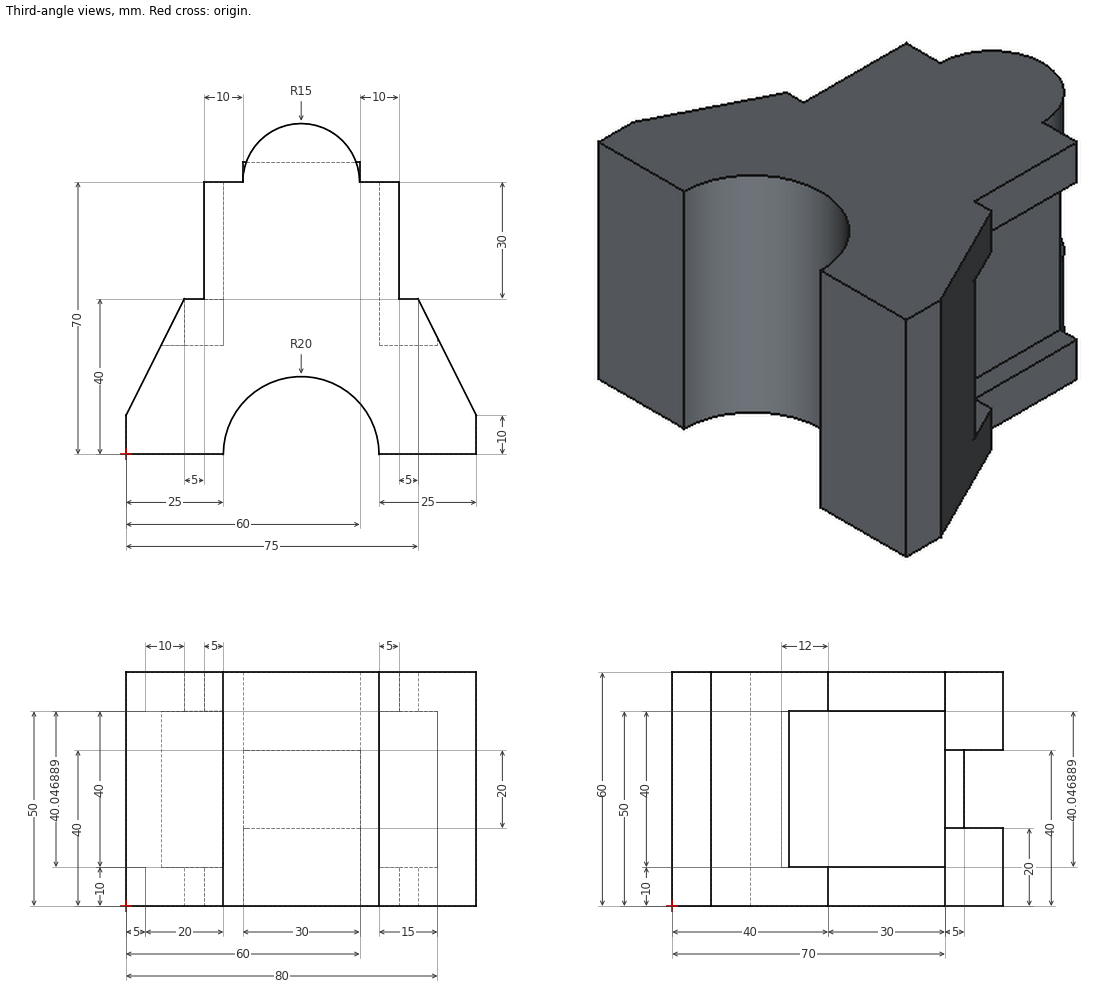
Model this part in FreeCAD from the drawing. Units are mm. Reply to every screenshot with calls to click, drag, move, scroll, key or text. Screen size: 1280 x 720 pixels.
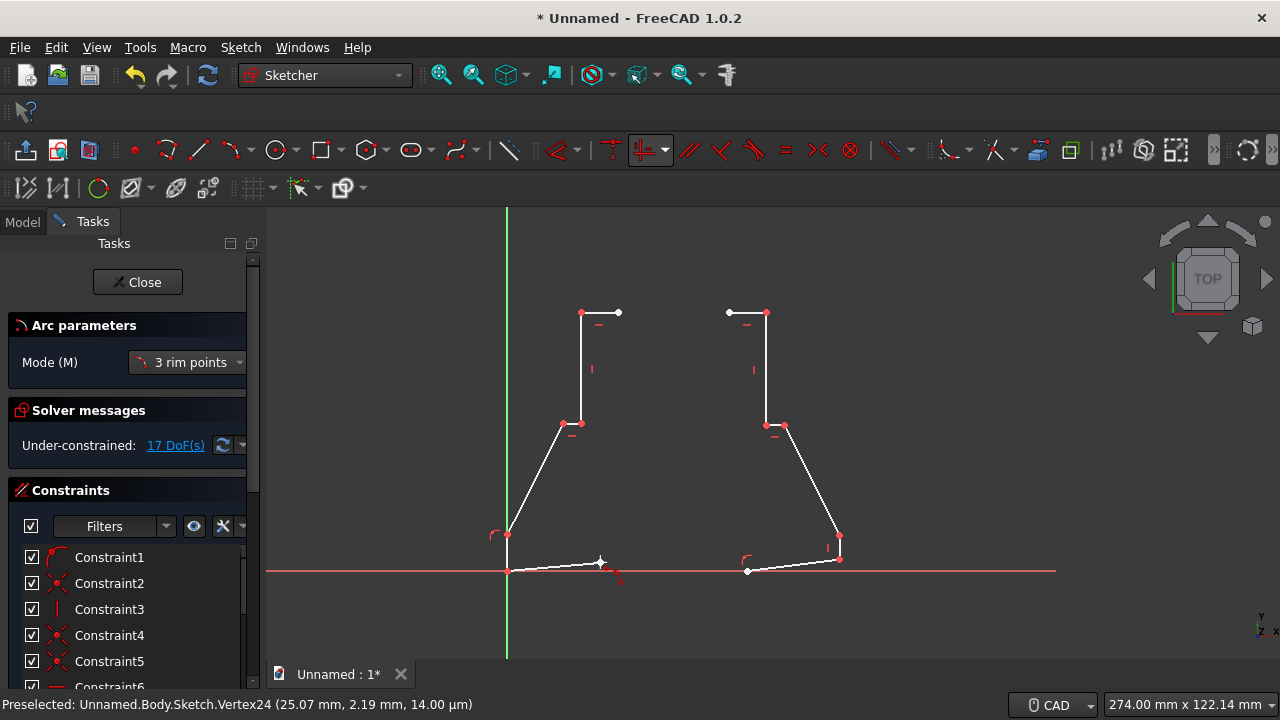
click(729, 313)
click(618, 313)
click(674, 257)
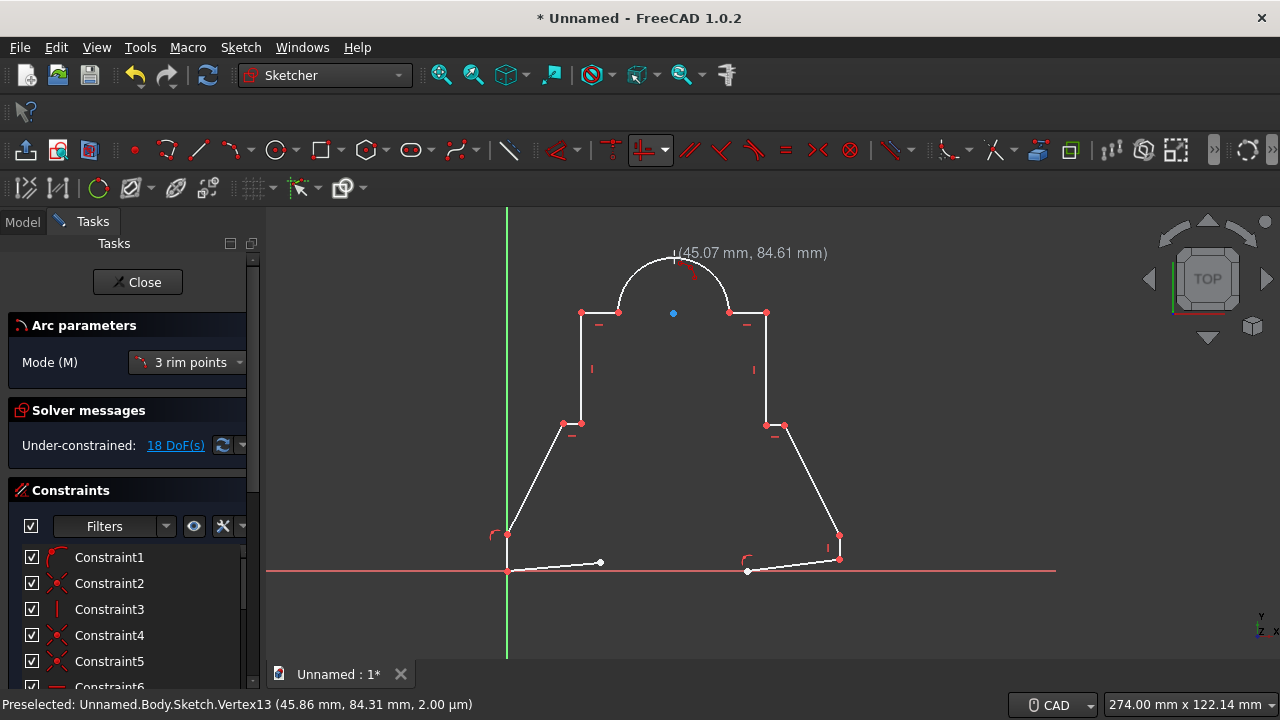
click(600, 563)
click(747, 571)
click(674, 497)
key(Escape)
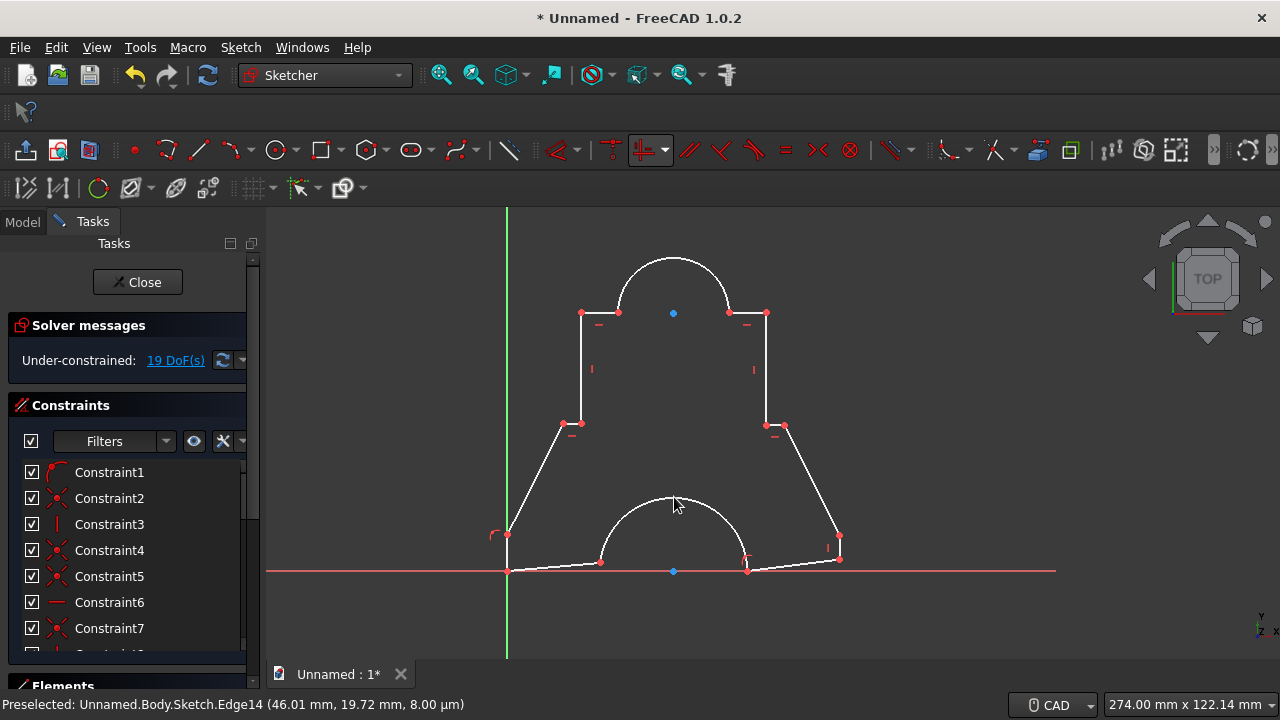
click(775, 568)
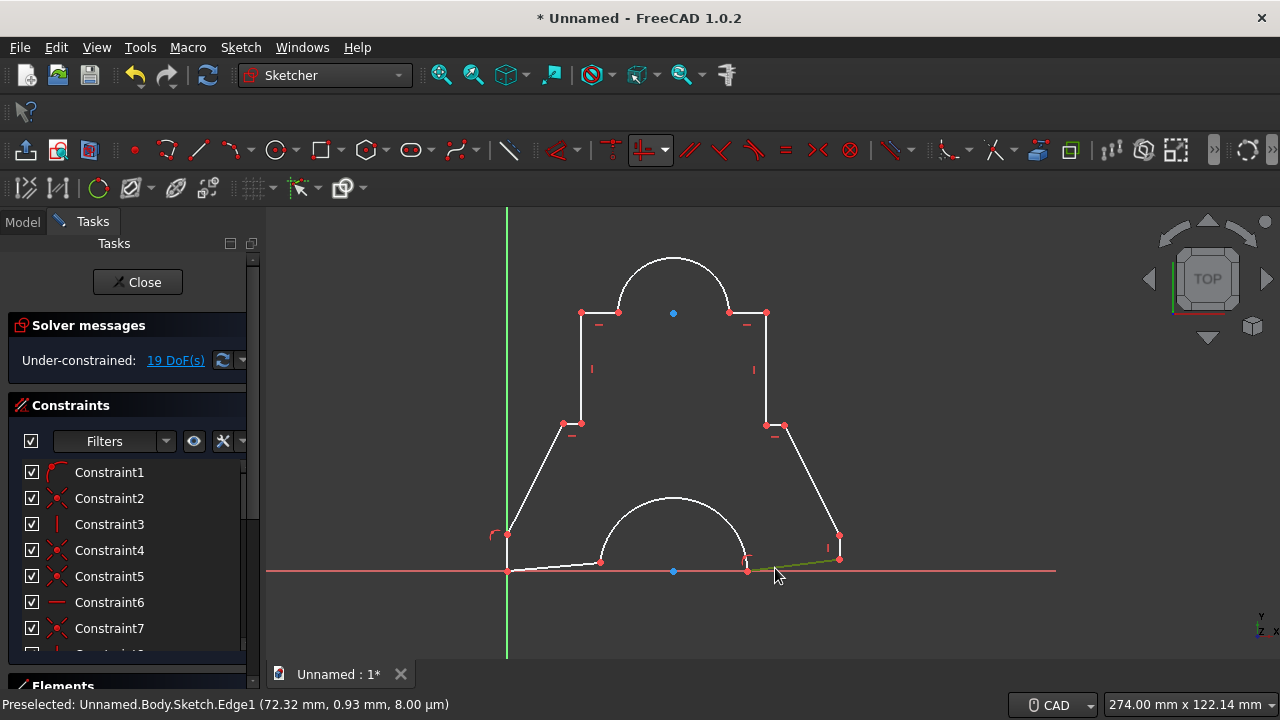
key(h)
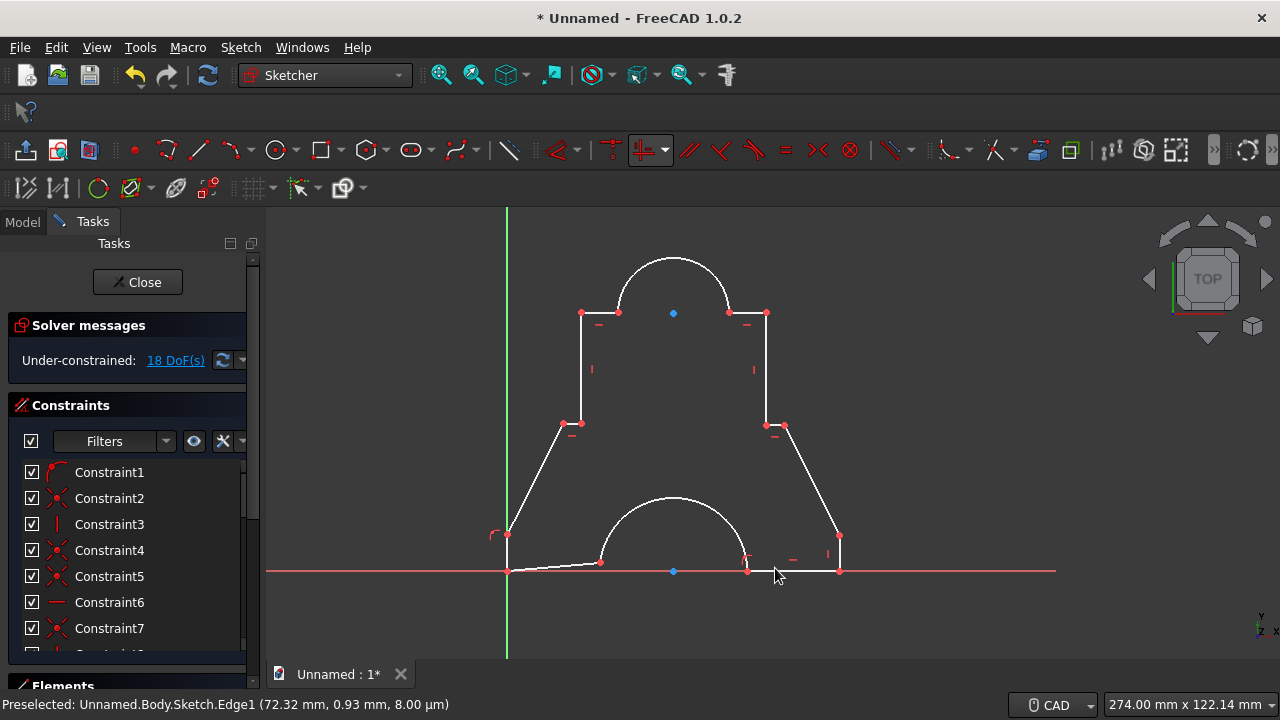
click(535, 569)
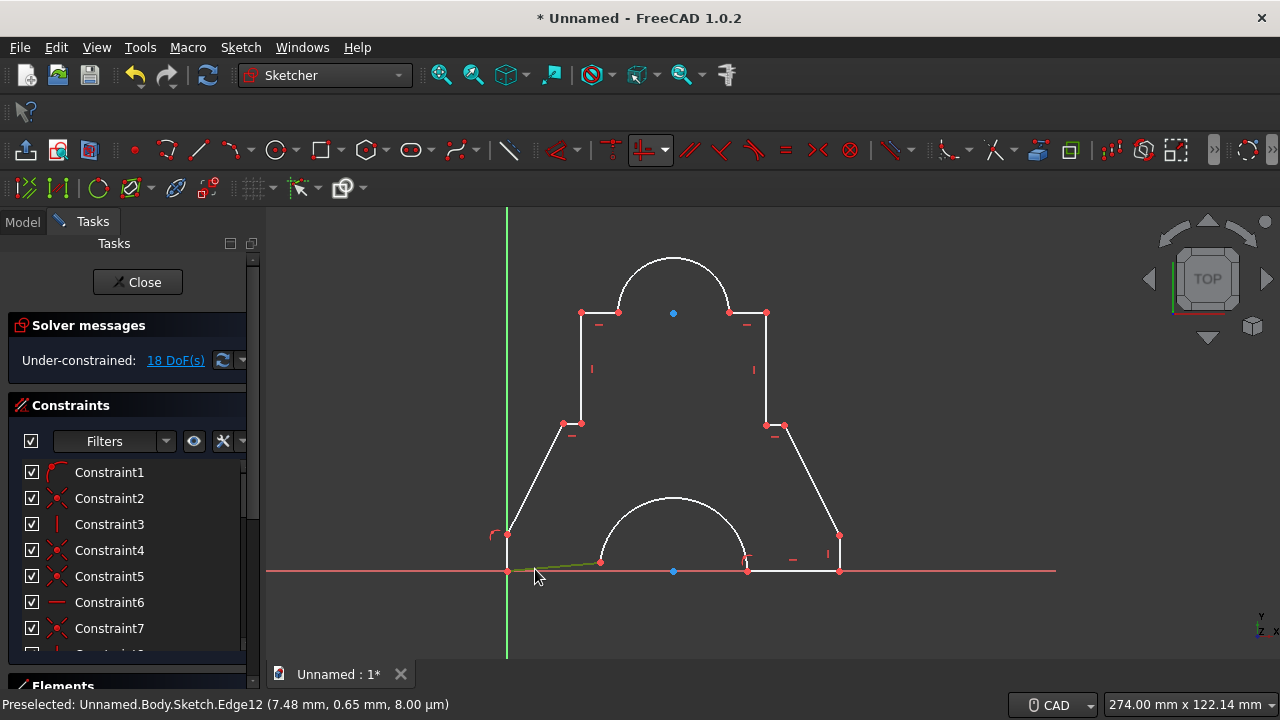
key(h)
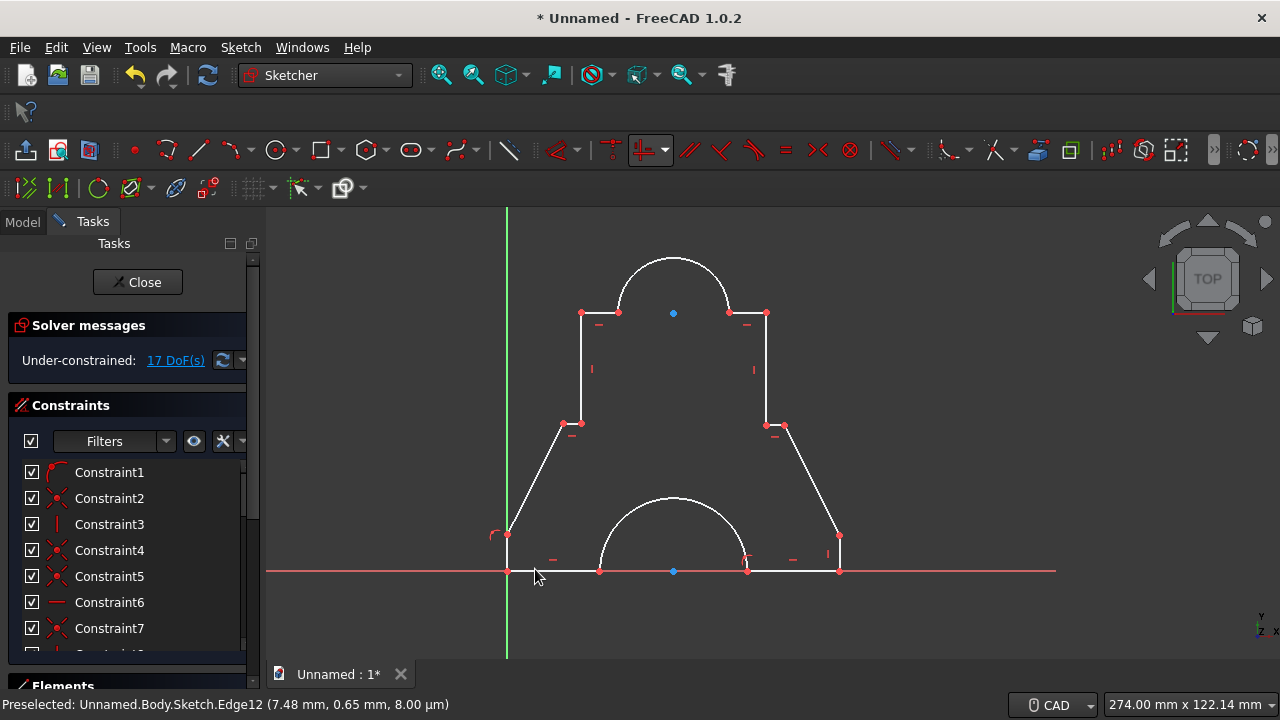
click(674, 572)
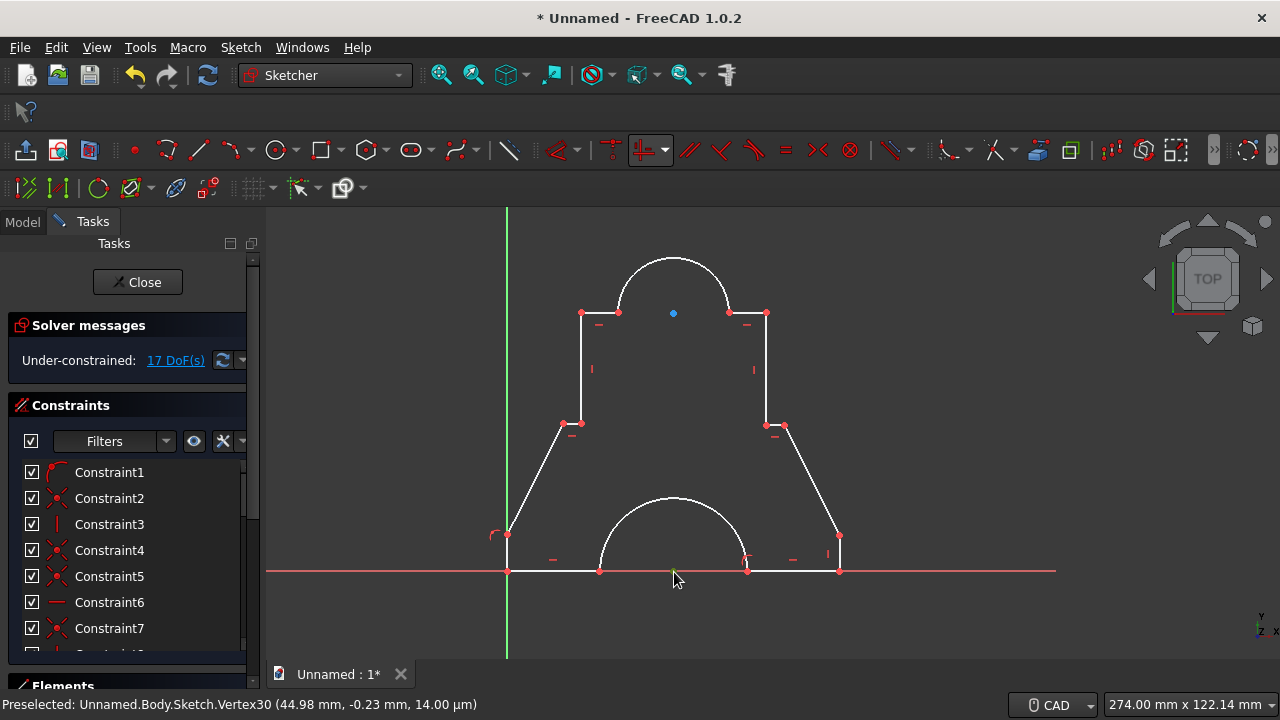
click(353, 571)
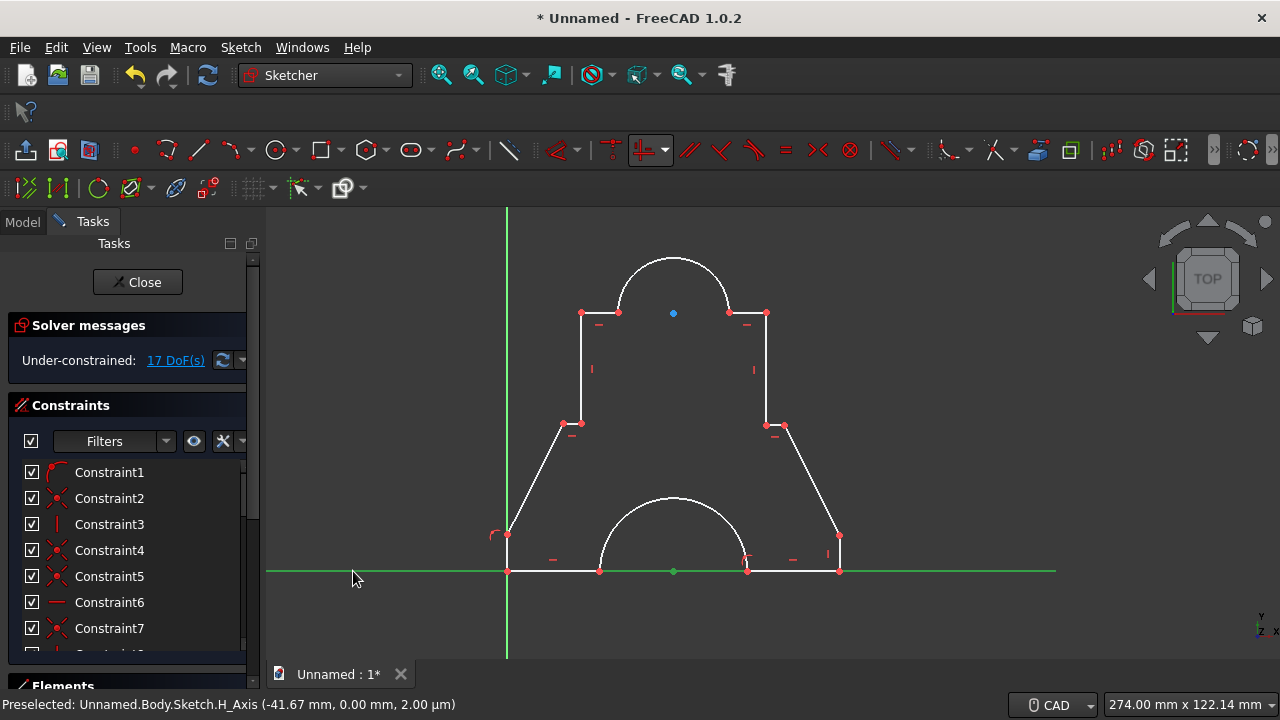
key(c)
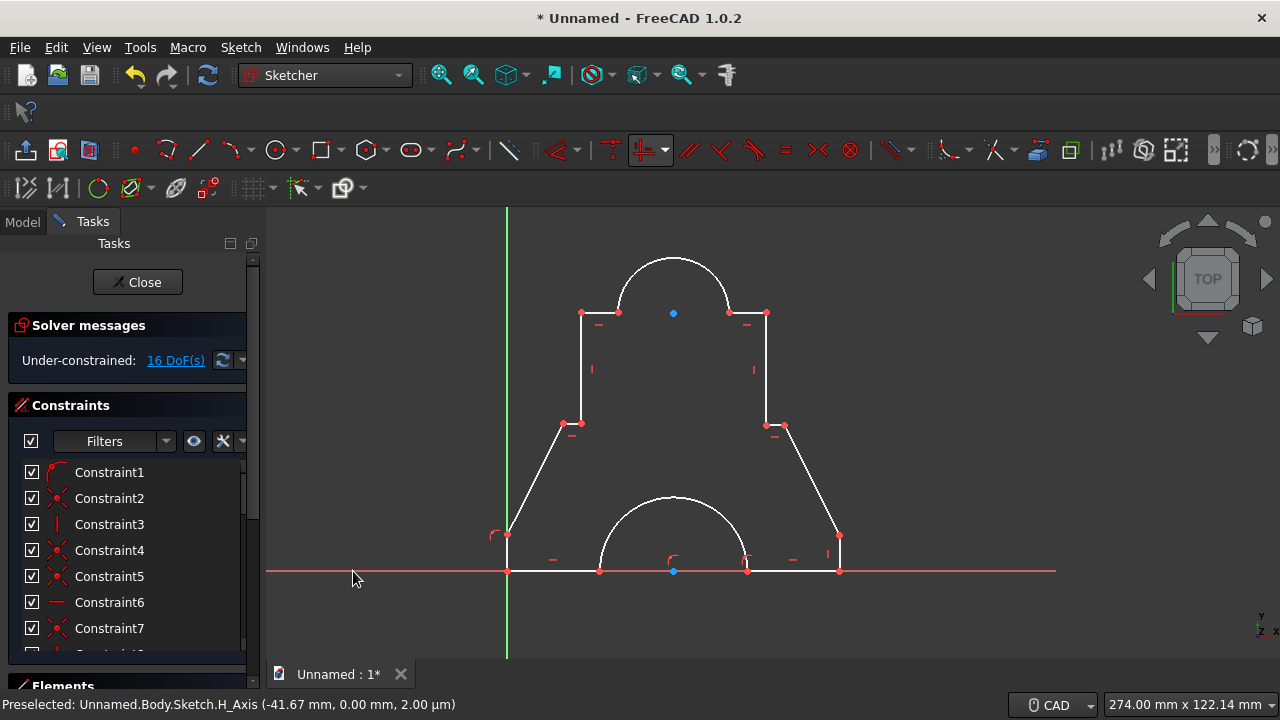
click(556, 150)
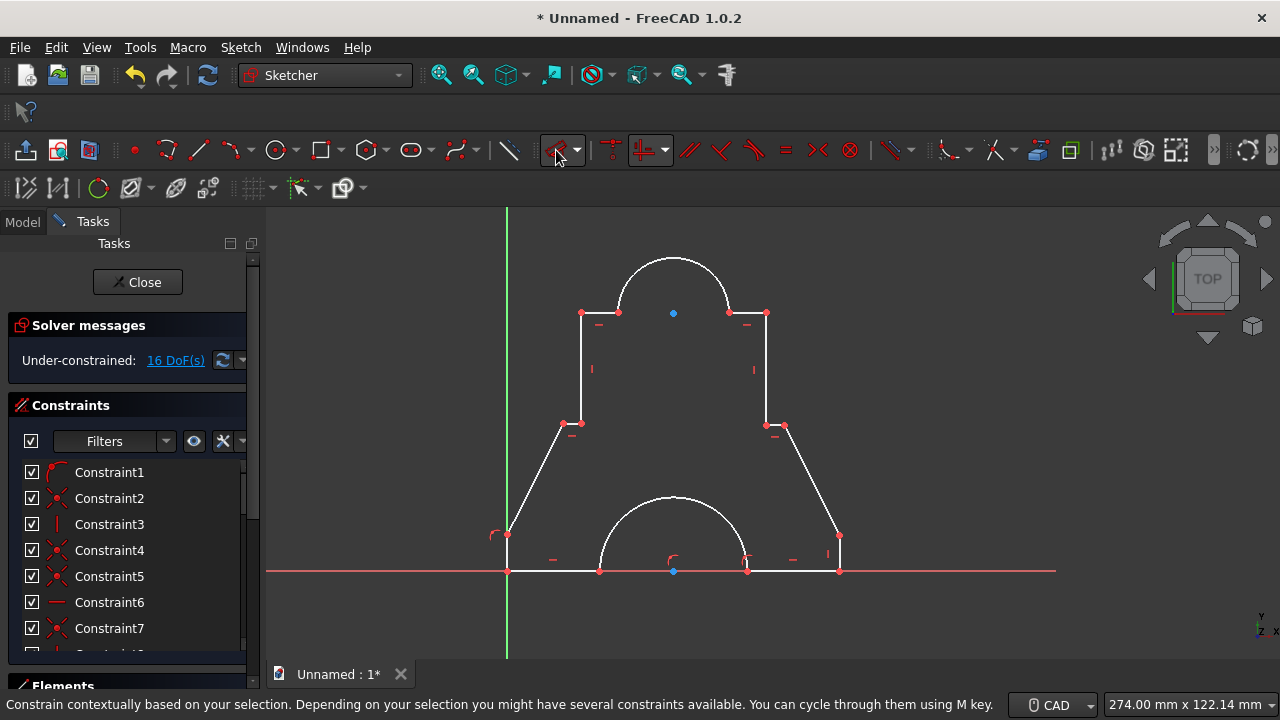
click(706, 268)
click(725, 242)